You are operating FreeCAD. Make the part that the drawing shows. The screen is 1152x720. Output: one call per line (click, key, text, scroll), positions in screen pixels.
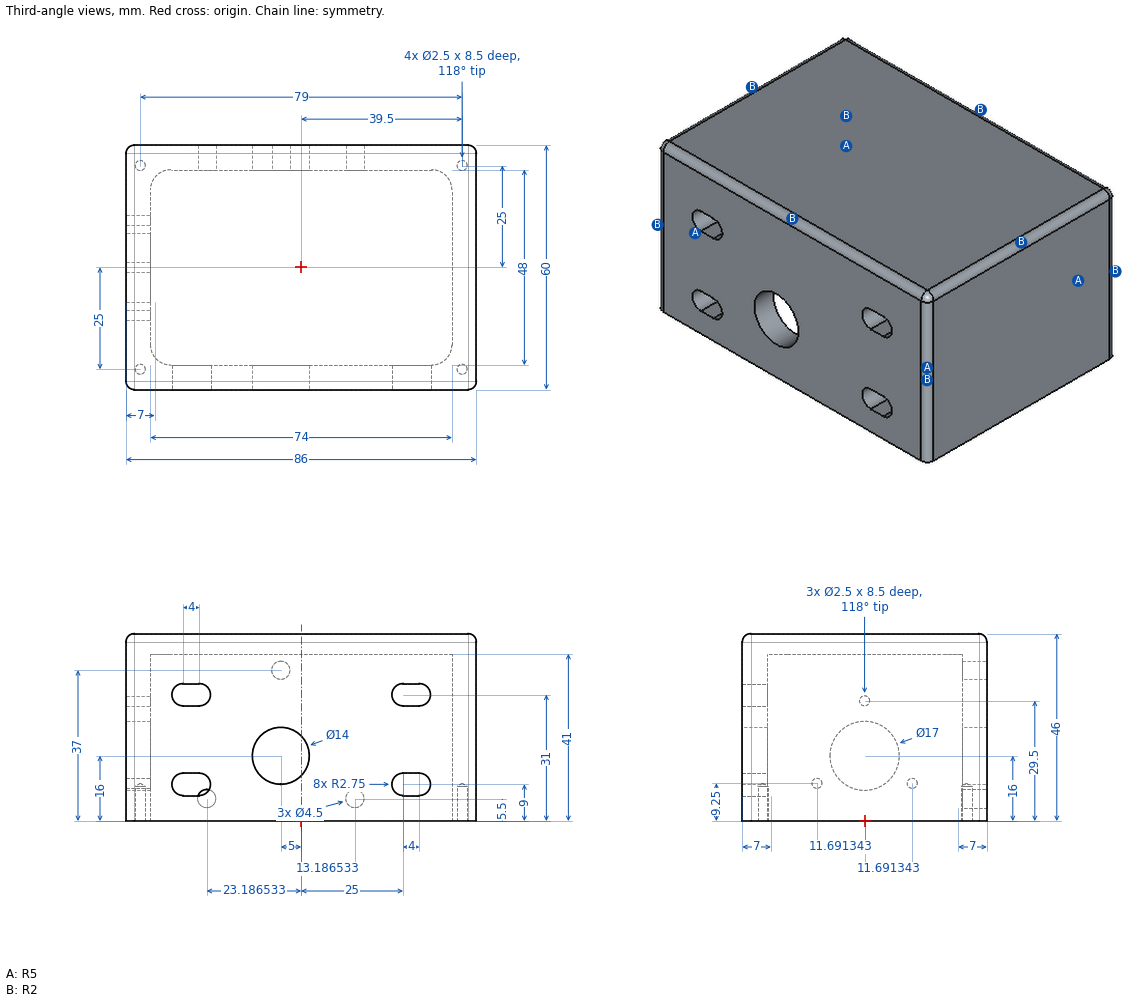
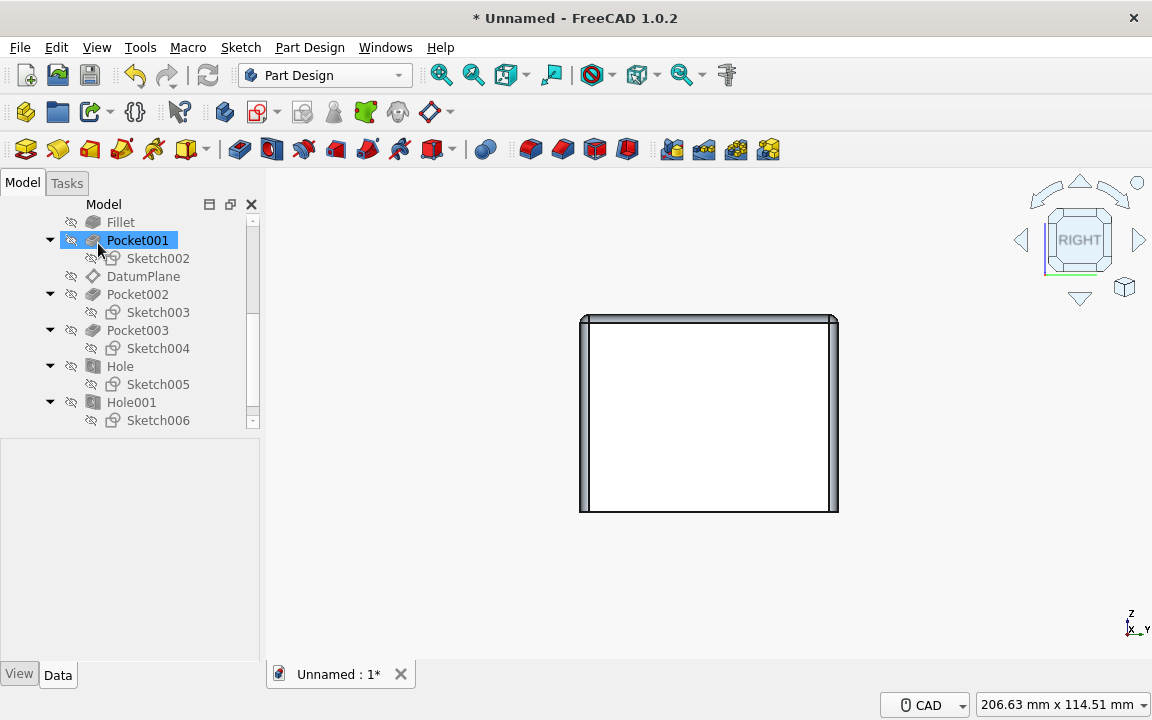
key(0)